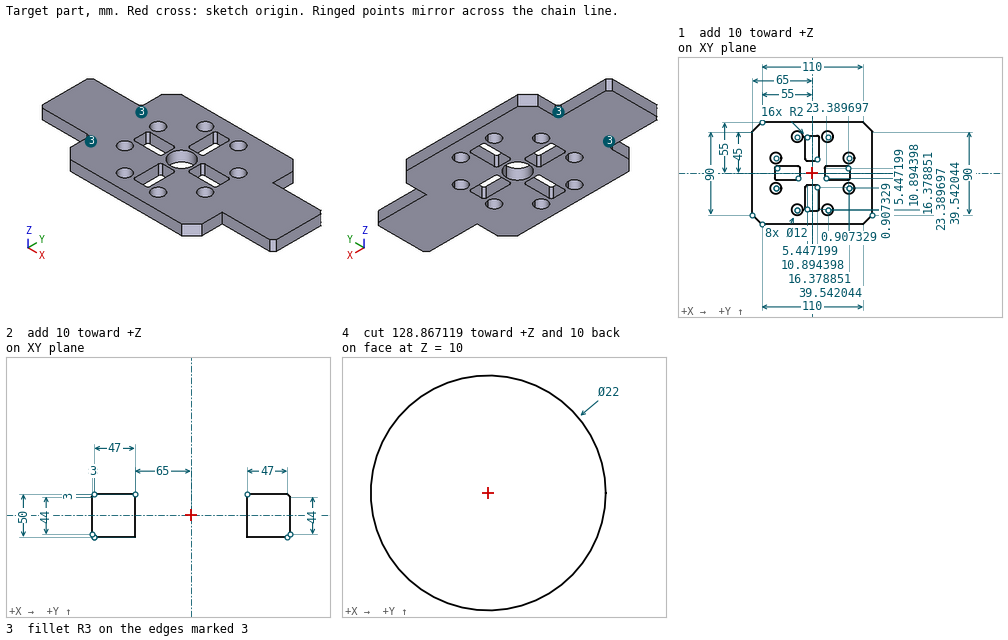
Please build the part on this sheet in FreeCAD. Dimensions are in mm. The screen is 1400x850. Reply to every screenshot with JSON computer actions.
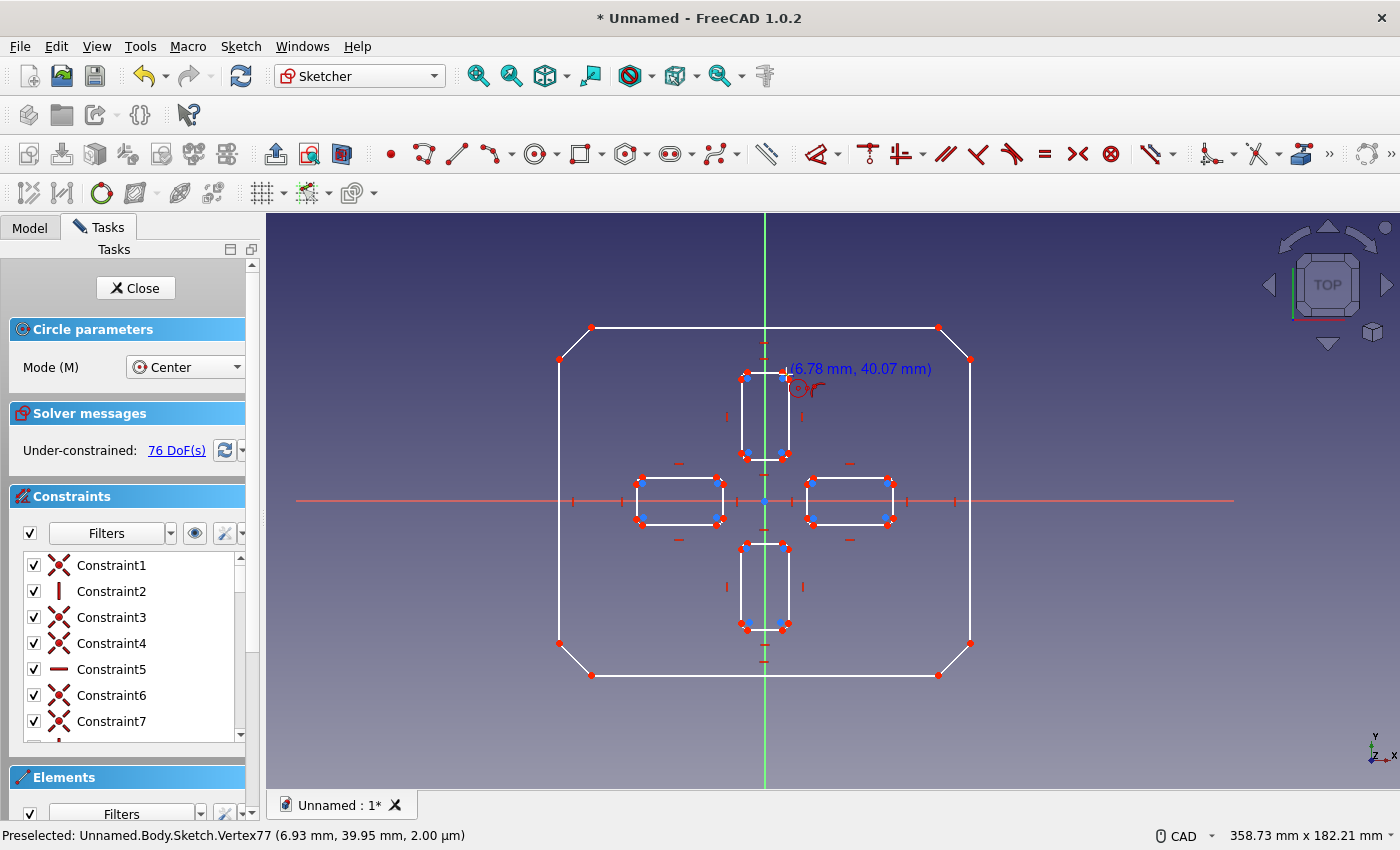
{"action": "left_click", "coordinate": [817, 626]}
{"action": "mouse_move", "coordinate": [830, 613]}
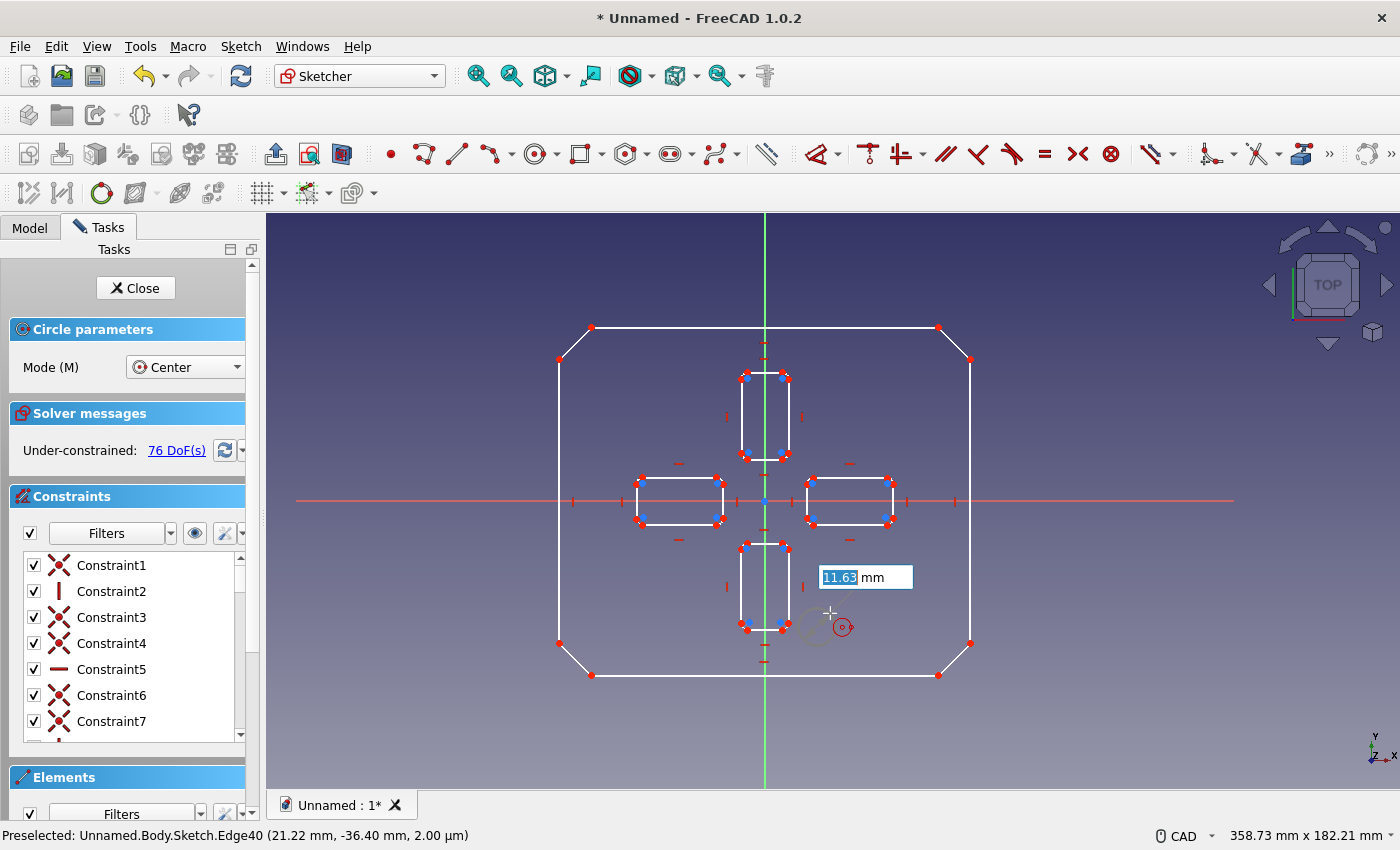
{"action": "type", "text": "12"}
{"action": "key", "text": "Return"}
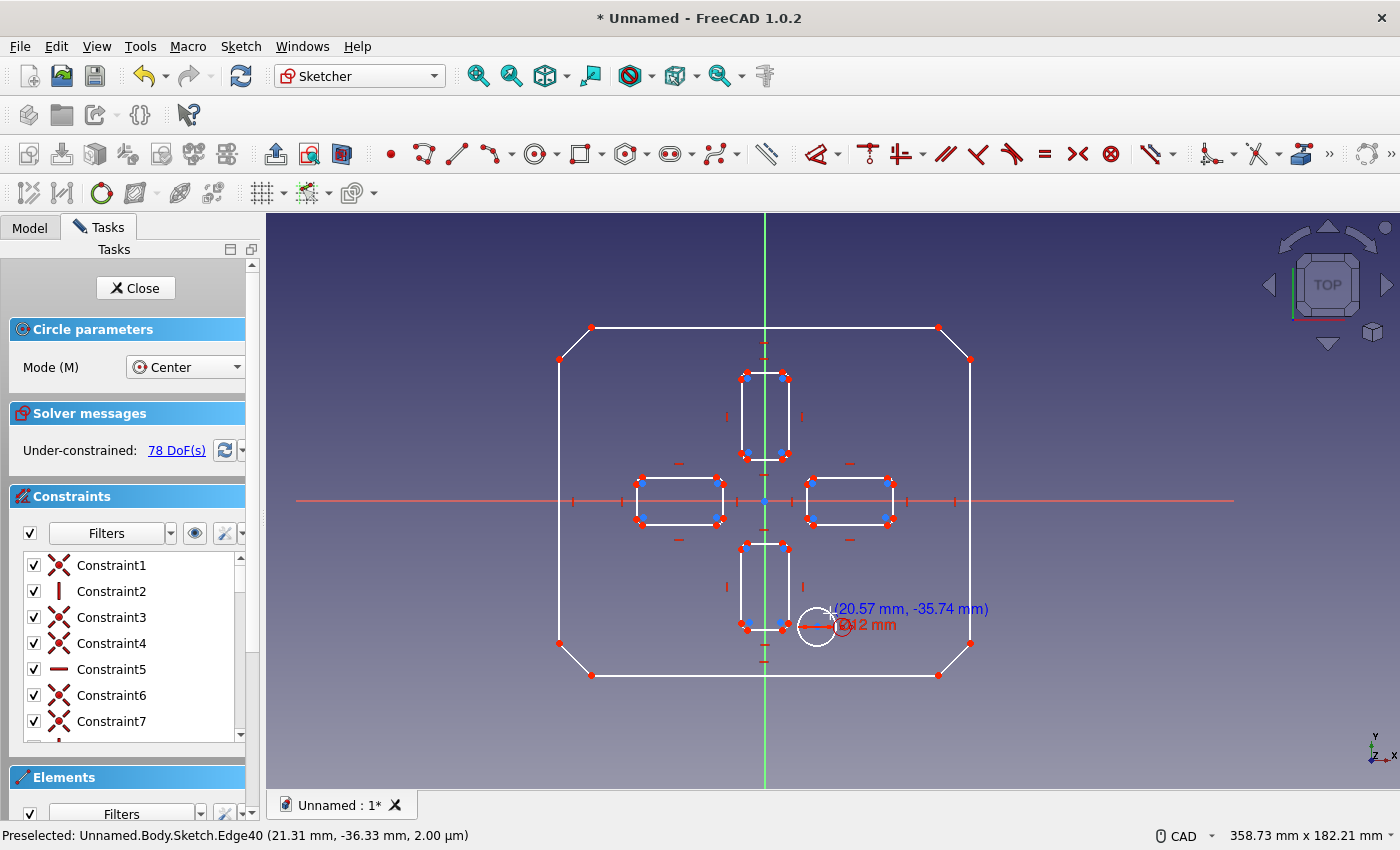
{"action": "left_click", "coordinate": [890, 553]}
{"action": "mouse_move", "coordinate": [903, 539]}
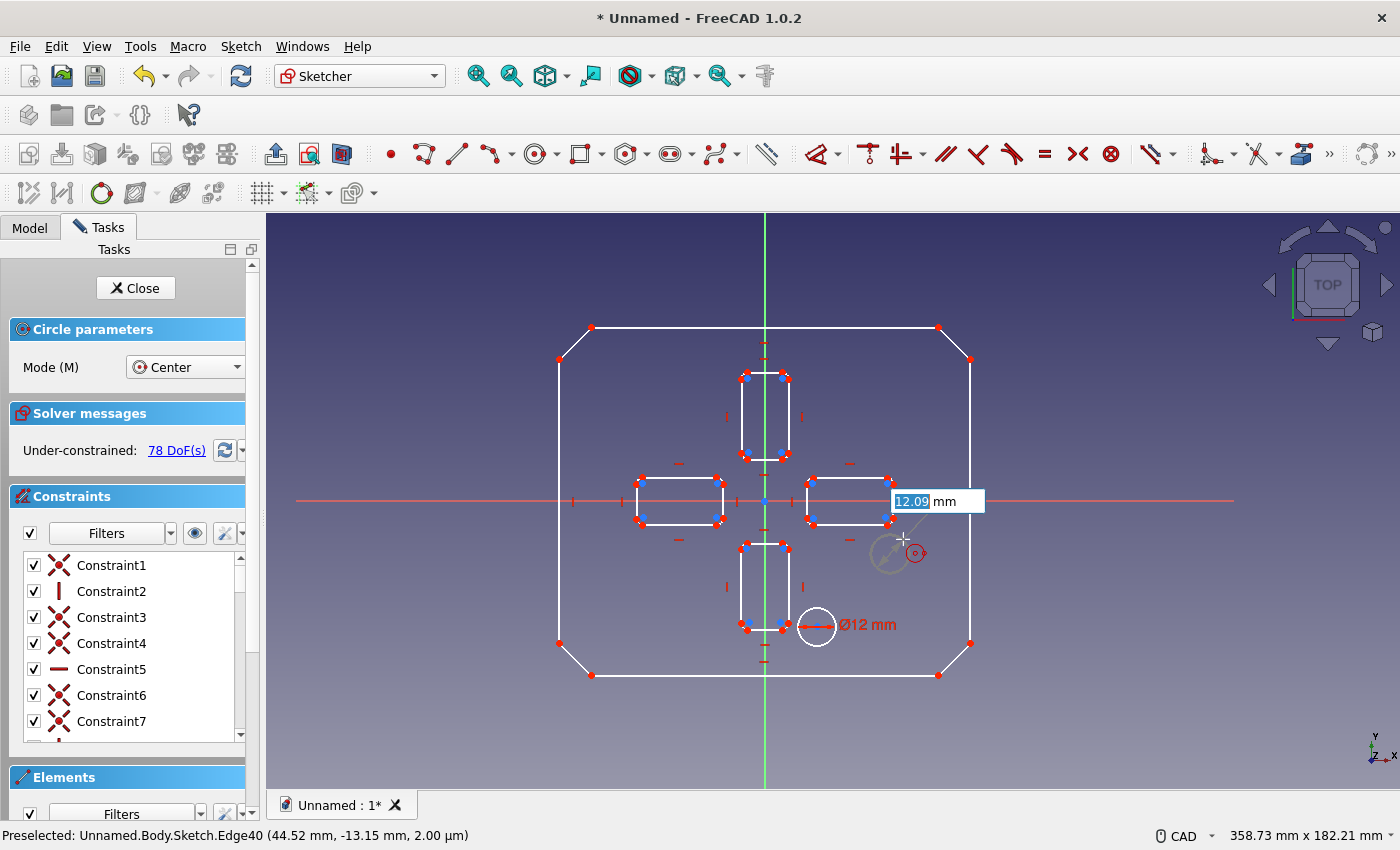
{"action": "type", "text": "12"}
{"action": "key", "text": "Return"}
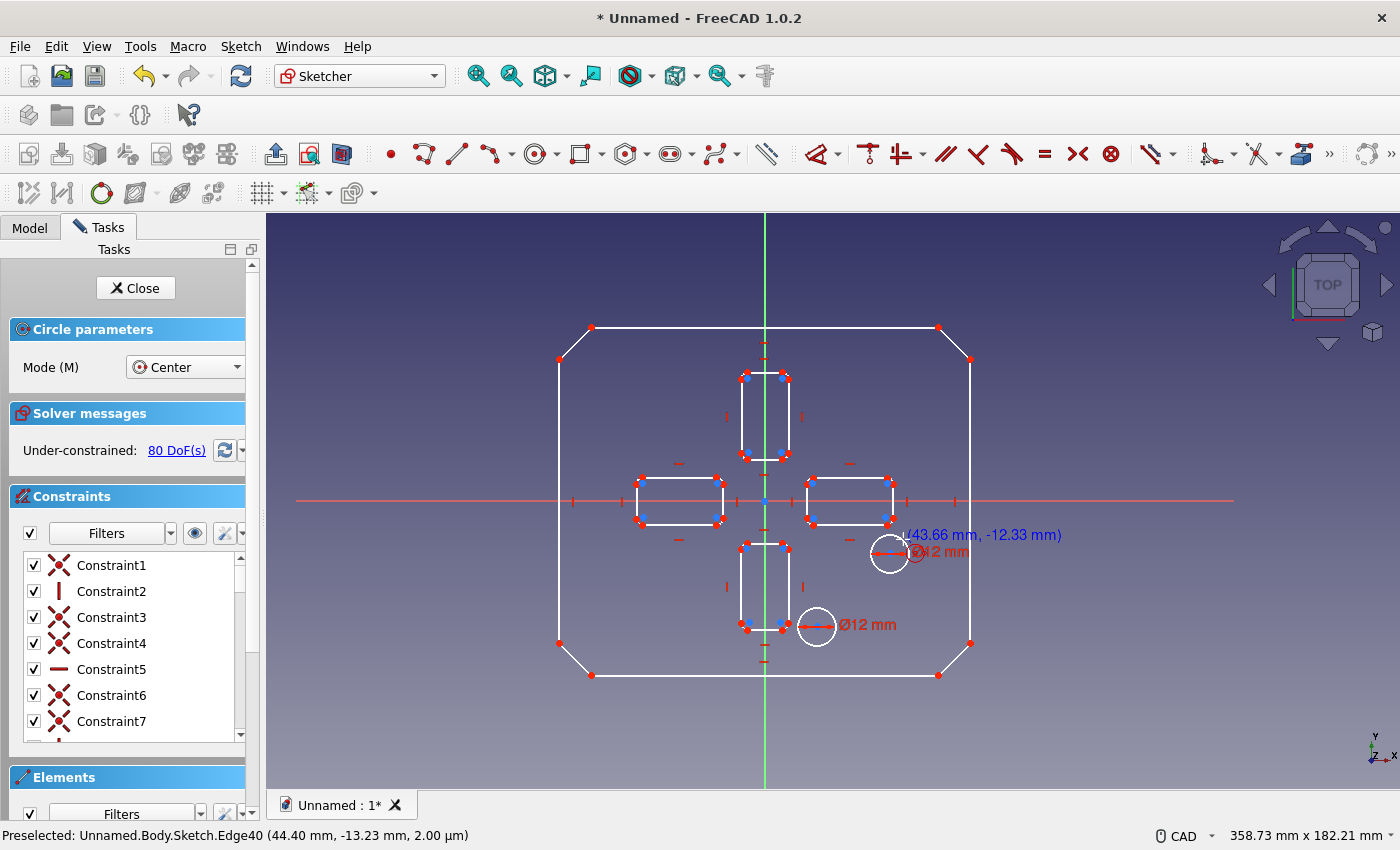
{"action": "left_click", "coordinate": [713, 626]}
{"action": "mouse_move", "coordinate": [727, 613]}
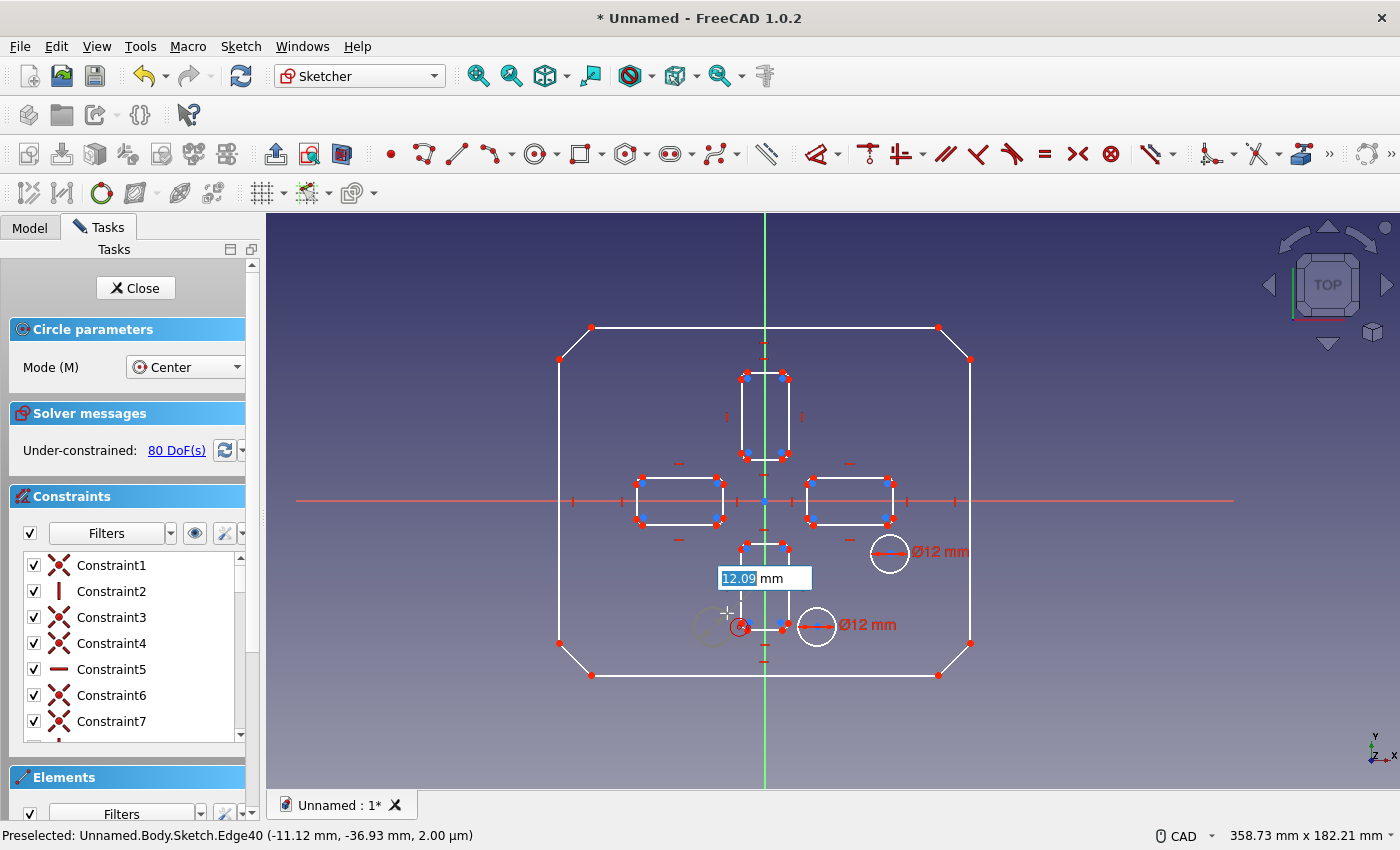
{"action": "type", "text": "12"}
{"action": "key", "text": "Return"}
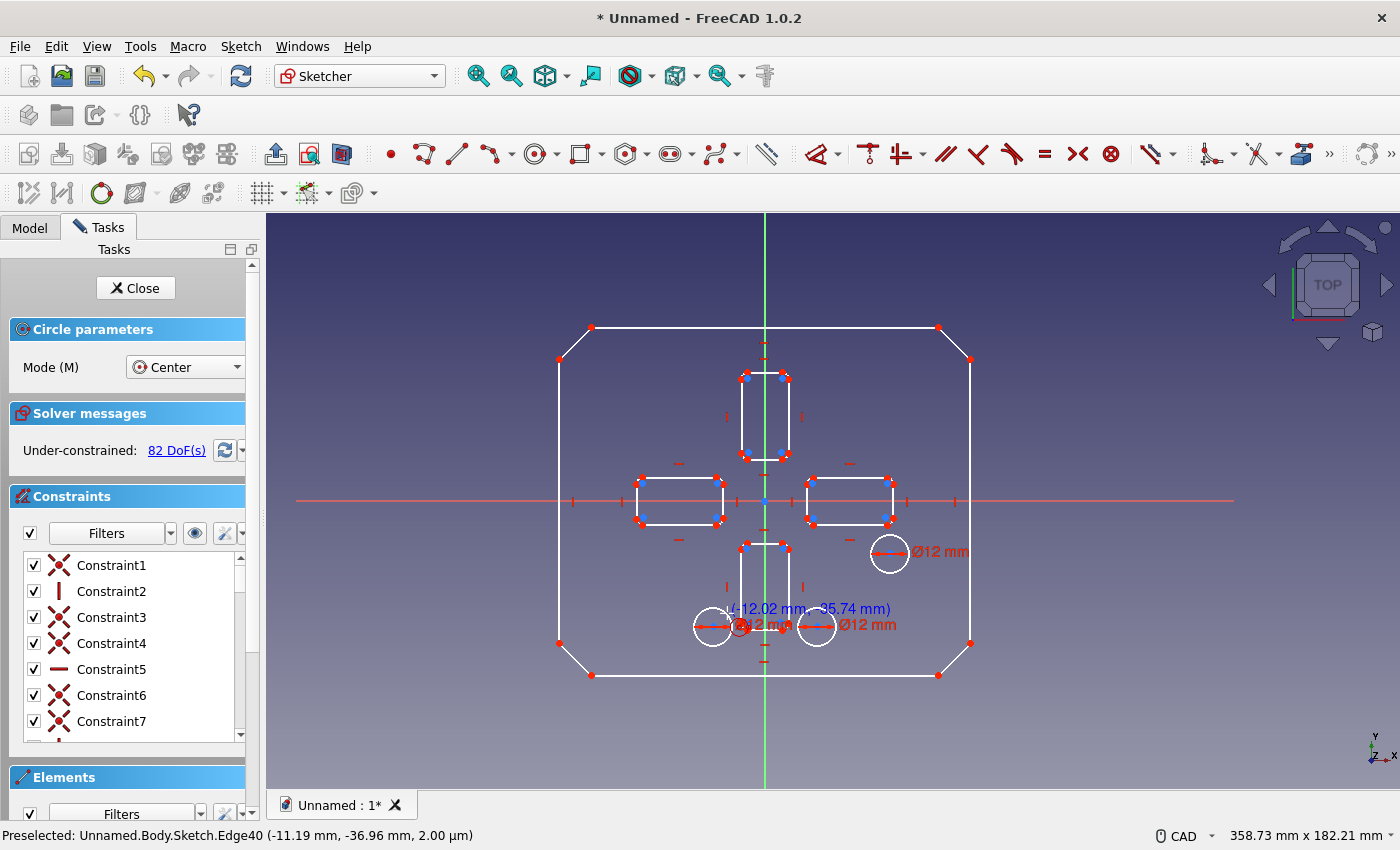
{"action": "left_click", "coordinate": [640, 553]}
{"action": "mouse_move", "coordinate": [653, 539]}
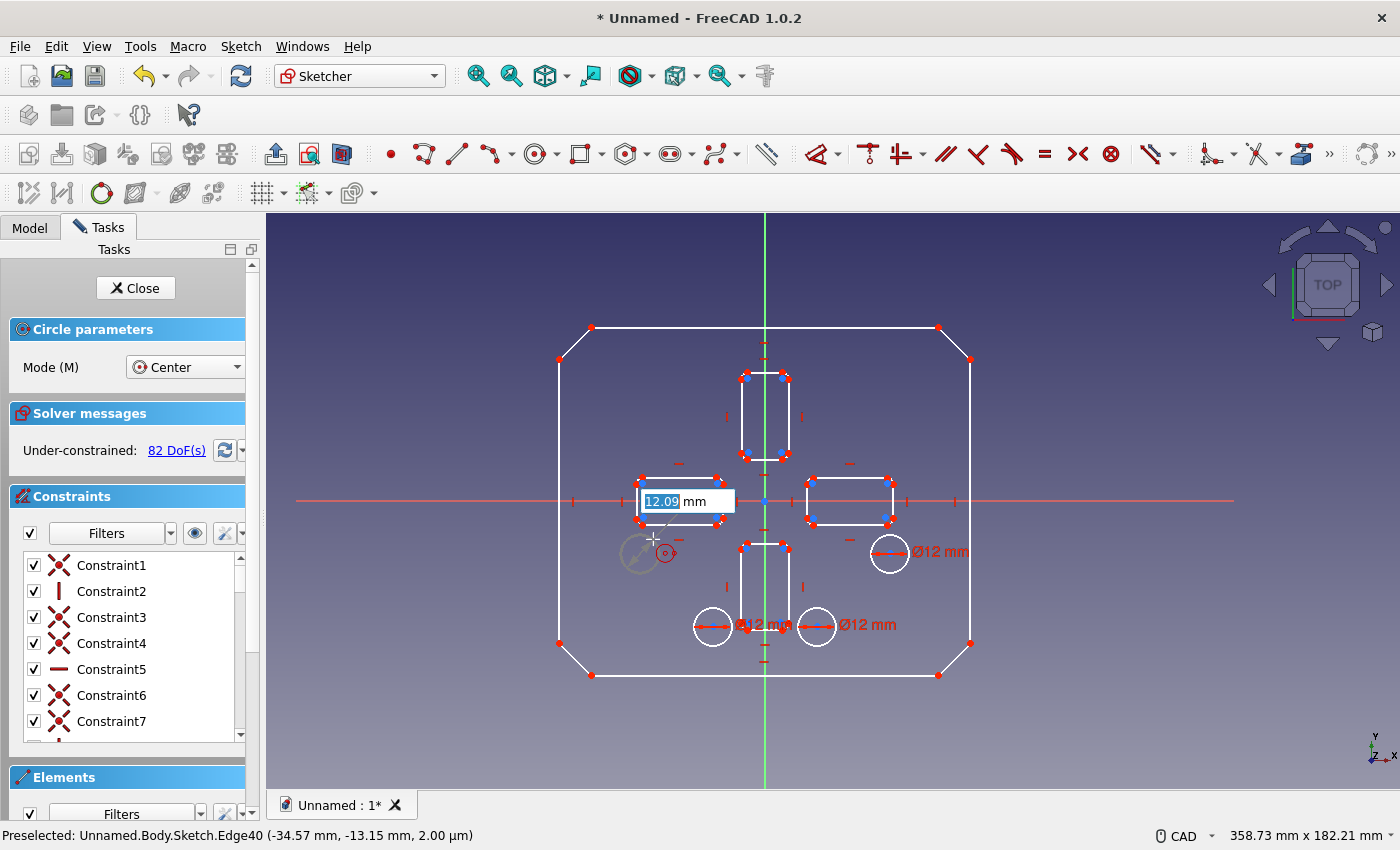
{"action": "type", "text": "12"}
{"action": "key", "text": "Return"}